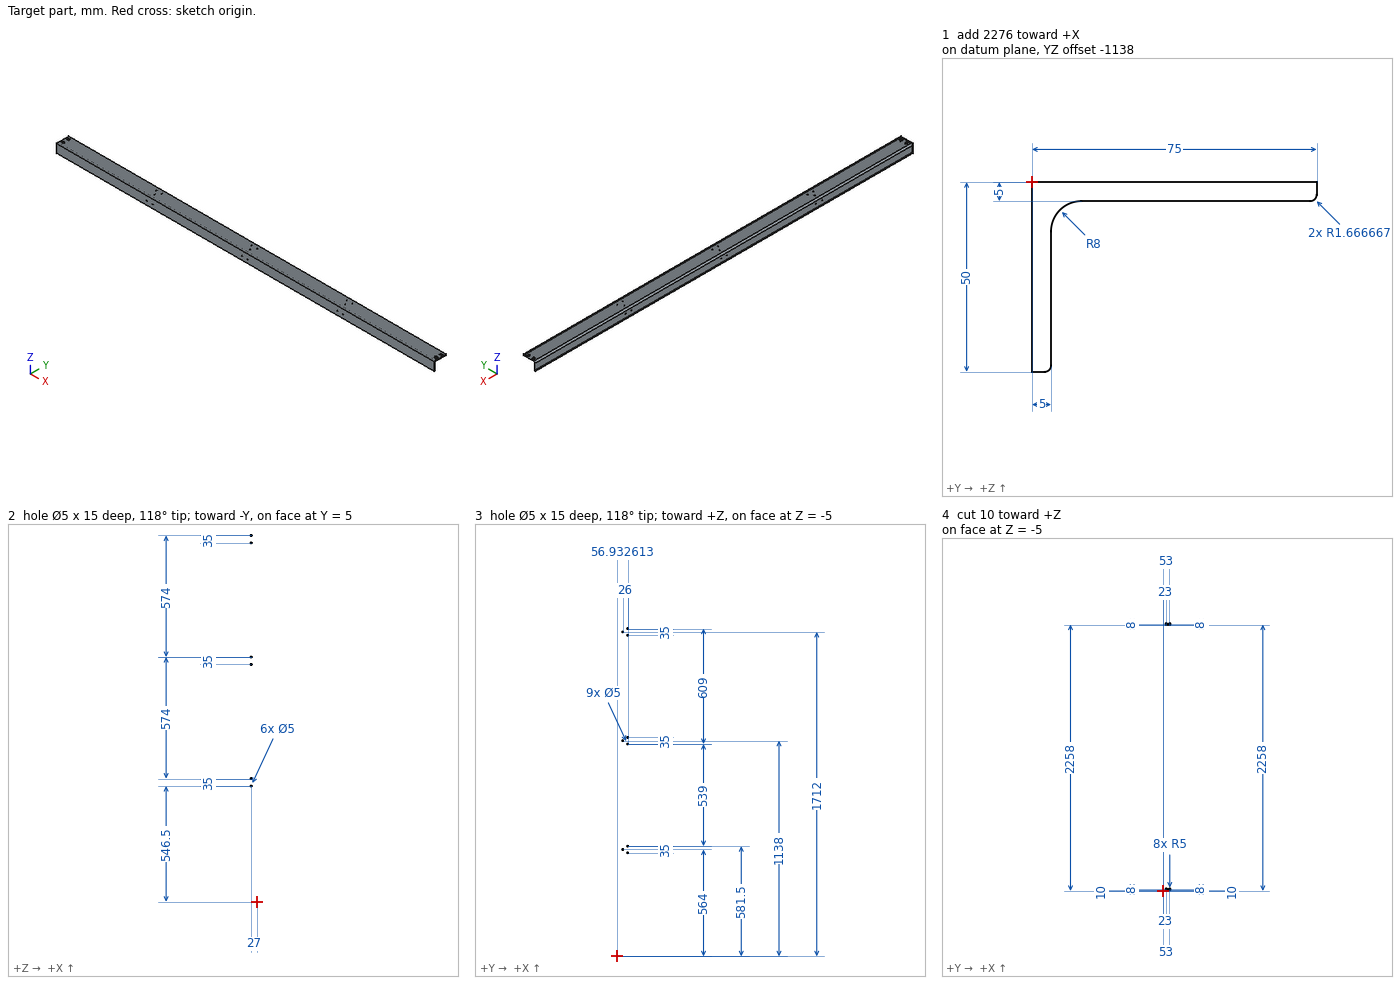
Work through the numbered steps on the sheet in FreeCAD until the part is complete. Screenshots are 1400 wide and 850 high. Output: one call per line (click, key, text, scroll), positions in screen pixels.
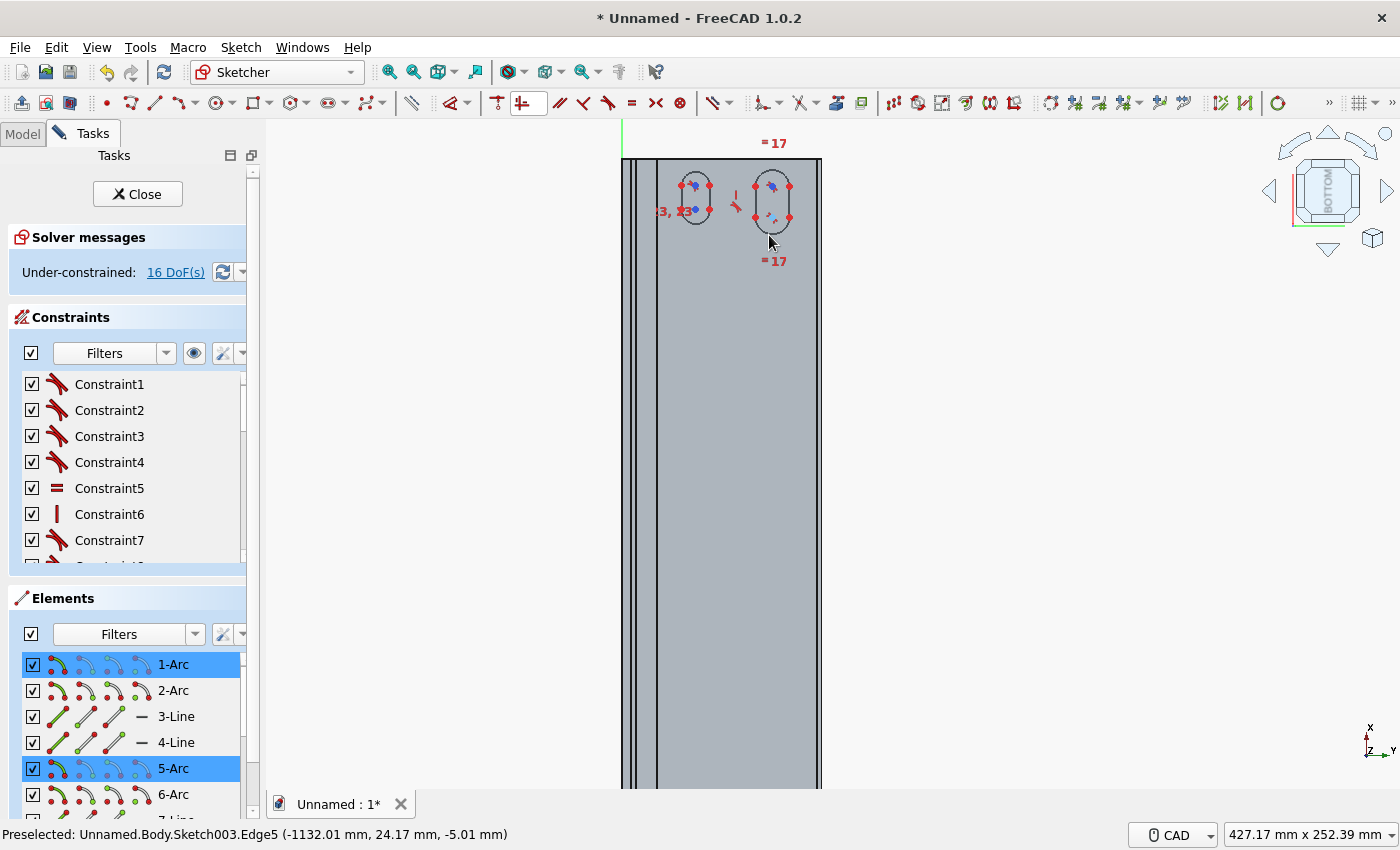
click(763, 231)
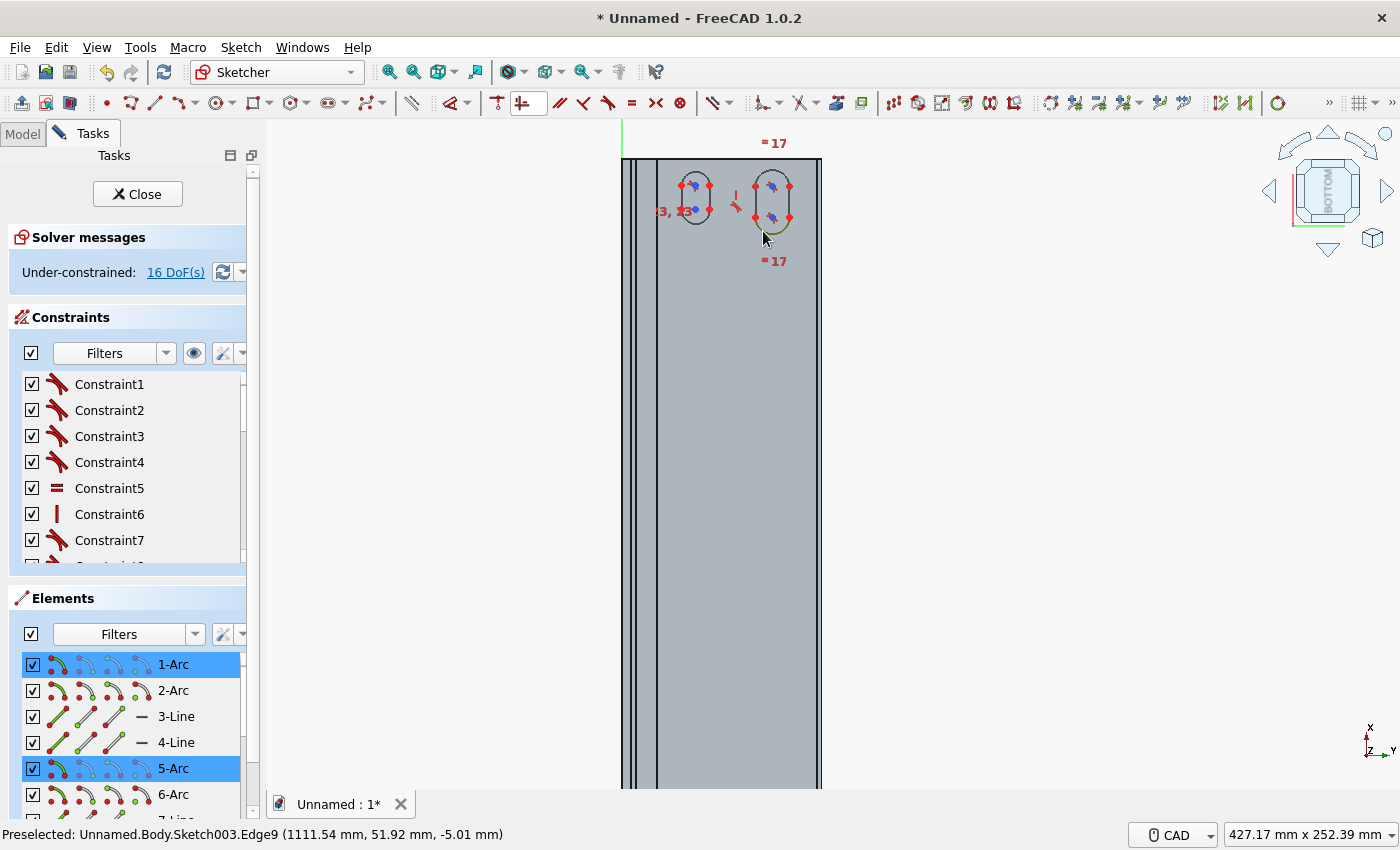
click(688, 221)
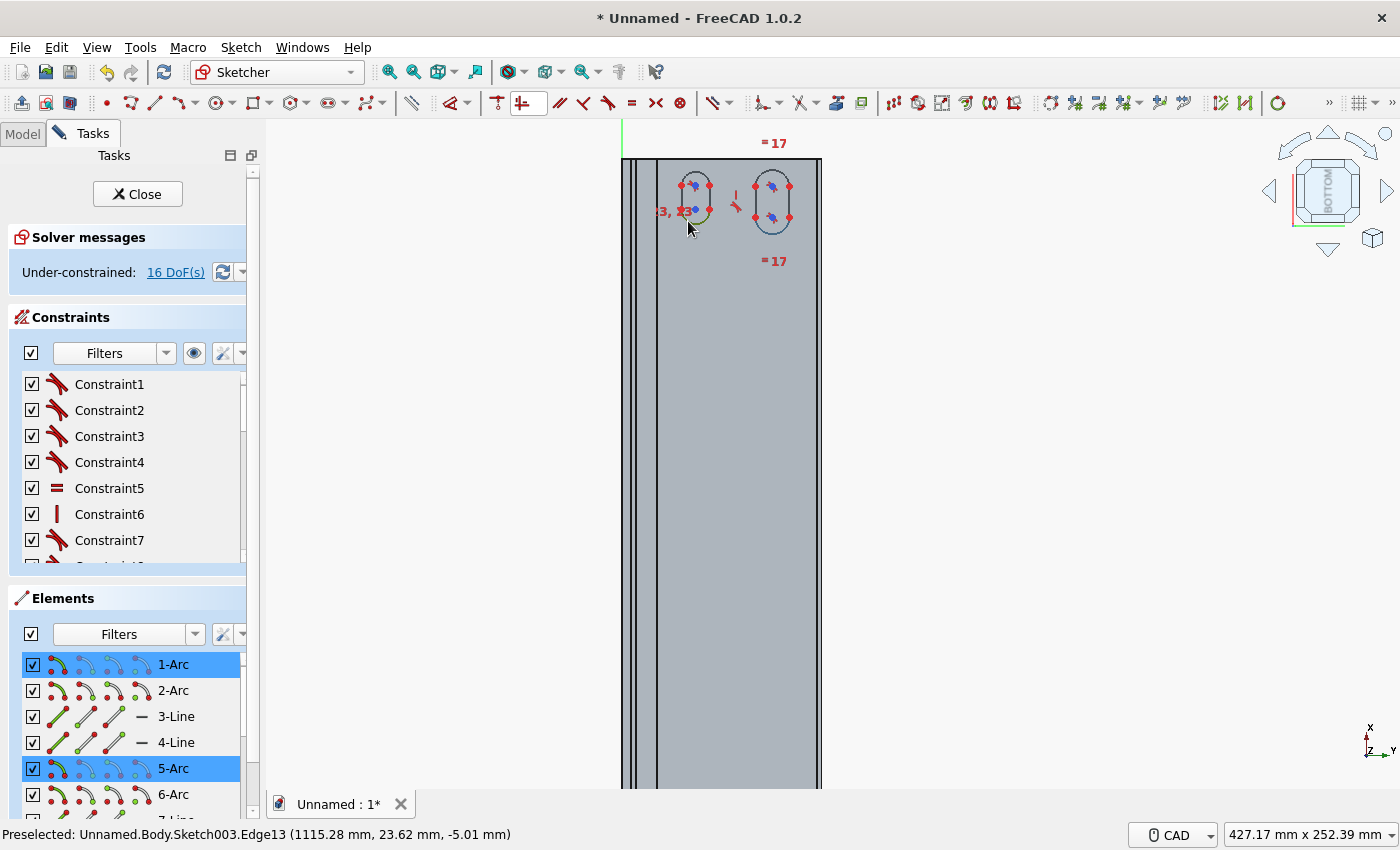
click(632, 104)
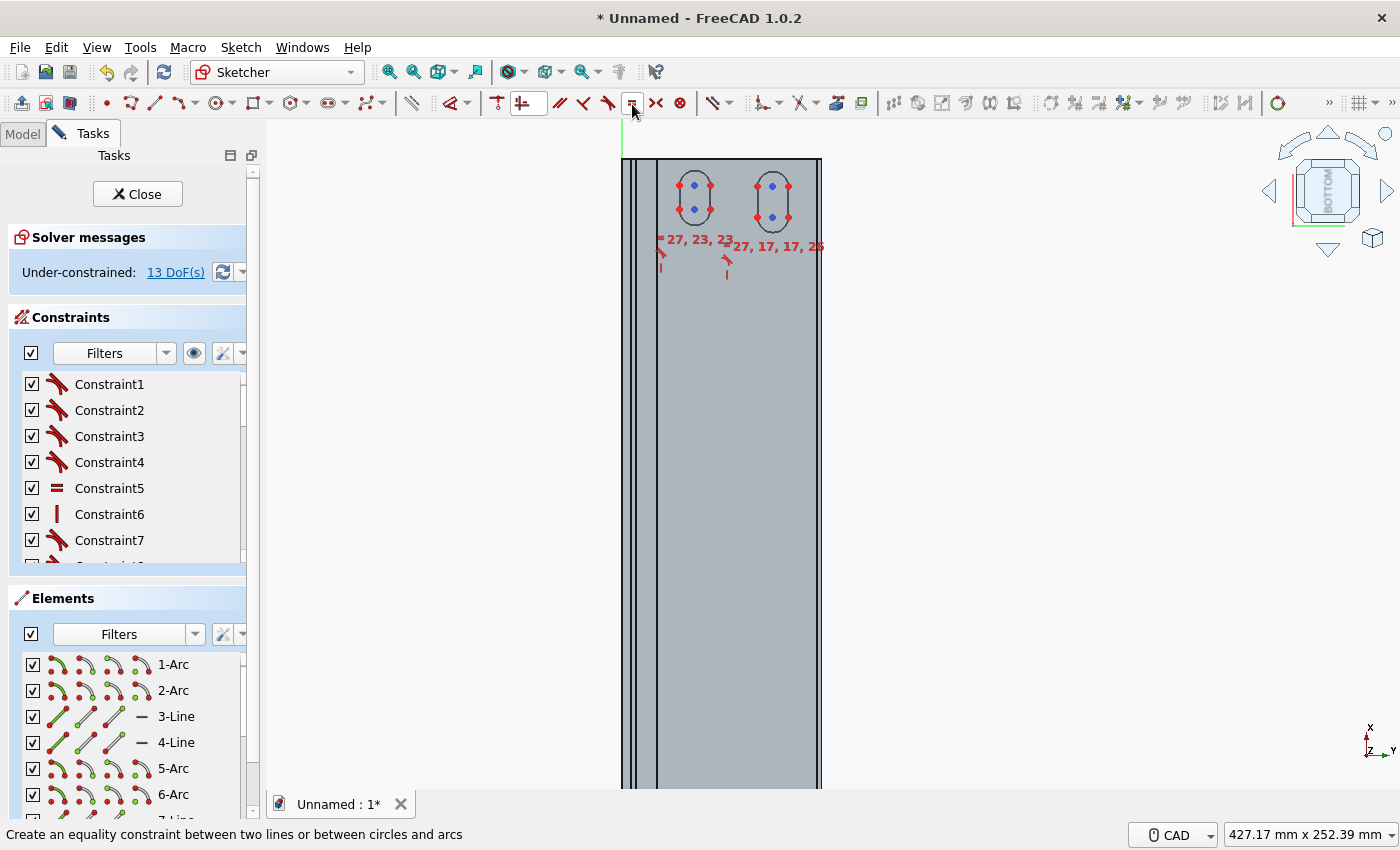
click(450, 104)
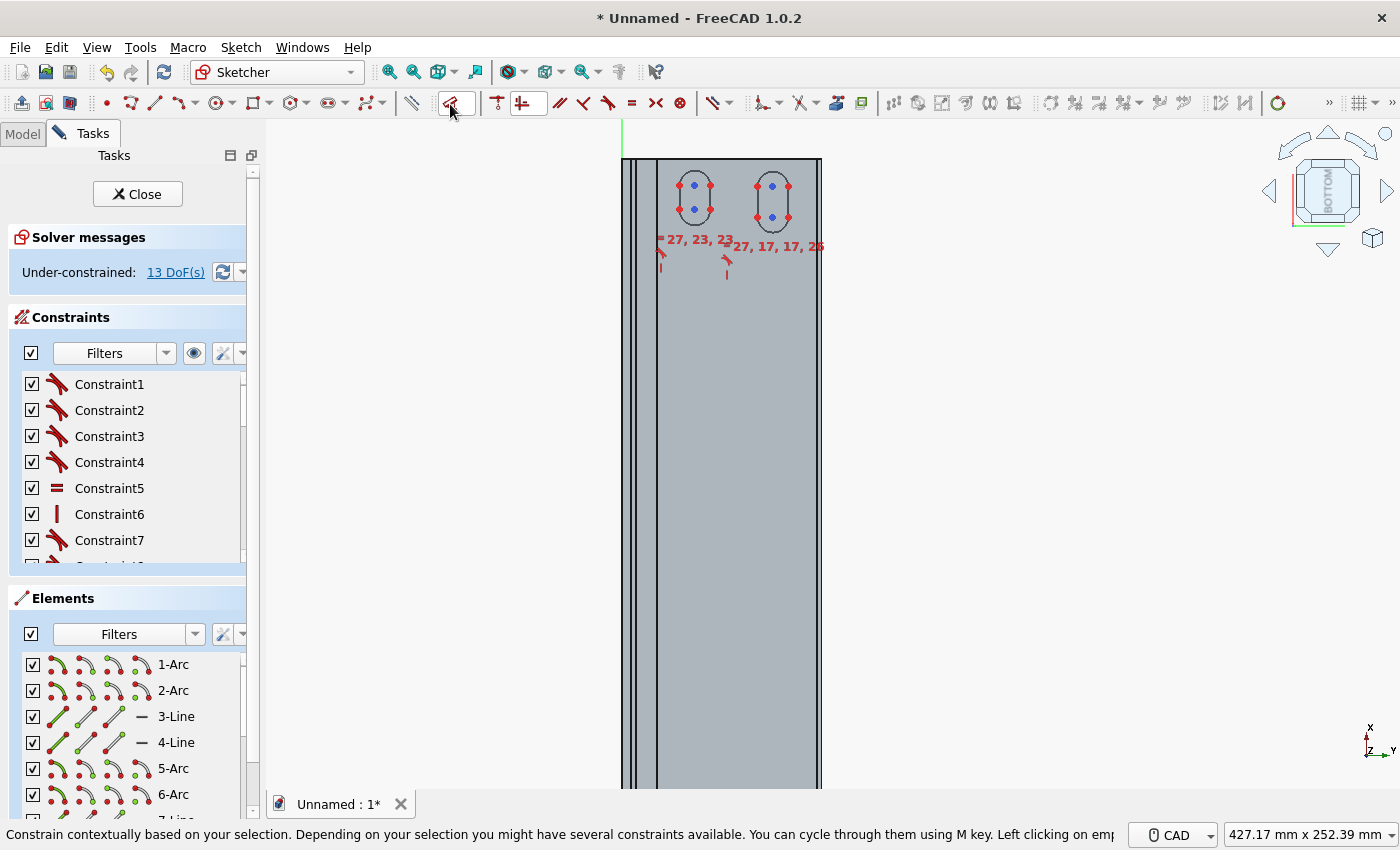
scroll(769, 235, down, 13)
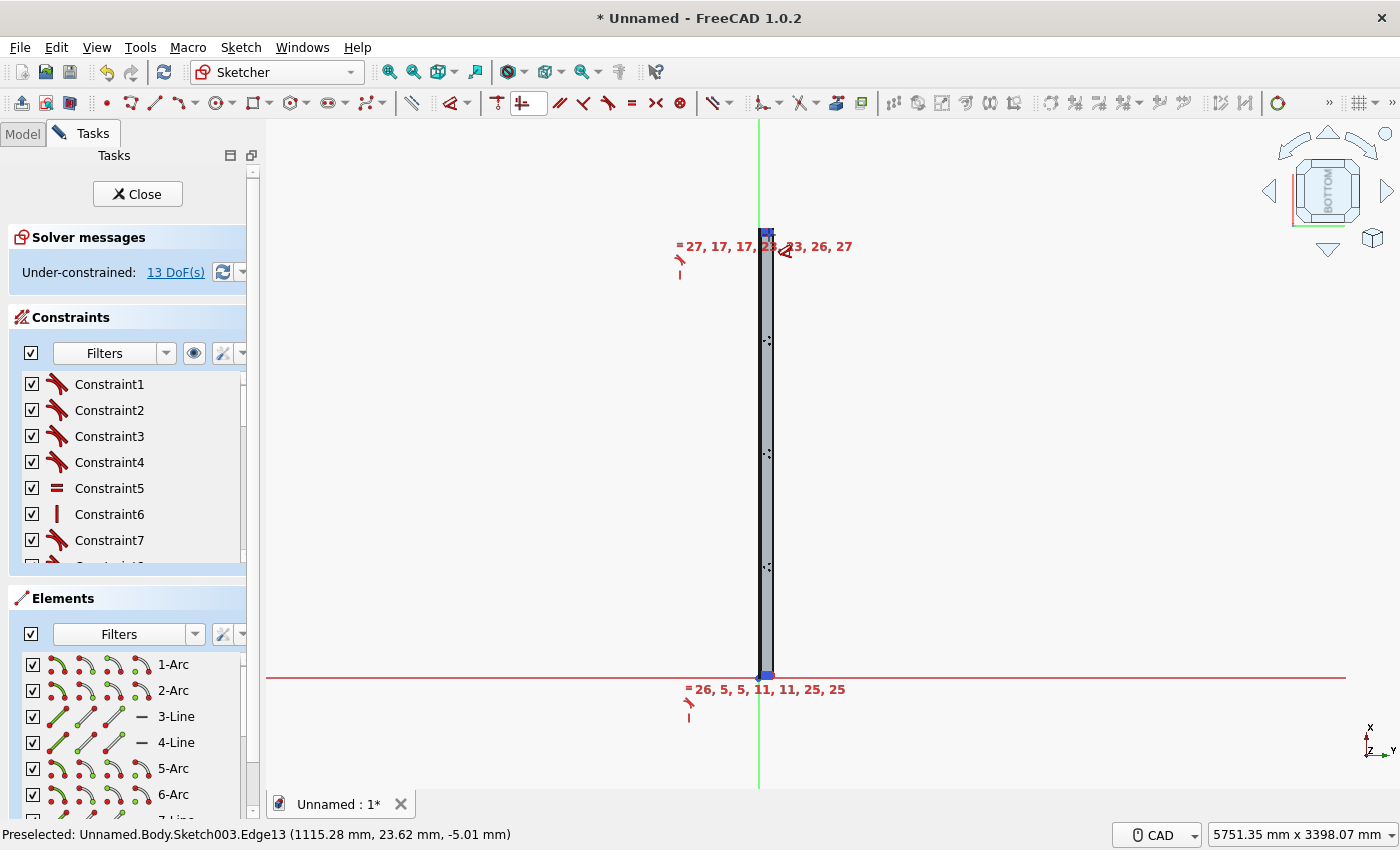
scroll(769, 677, up, 19)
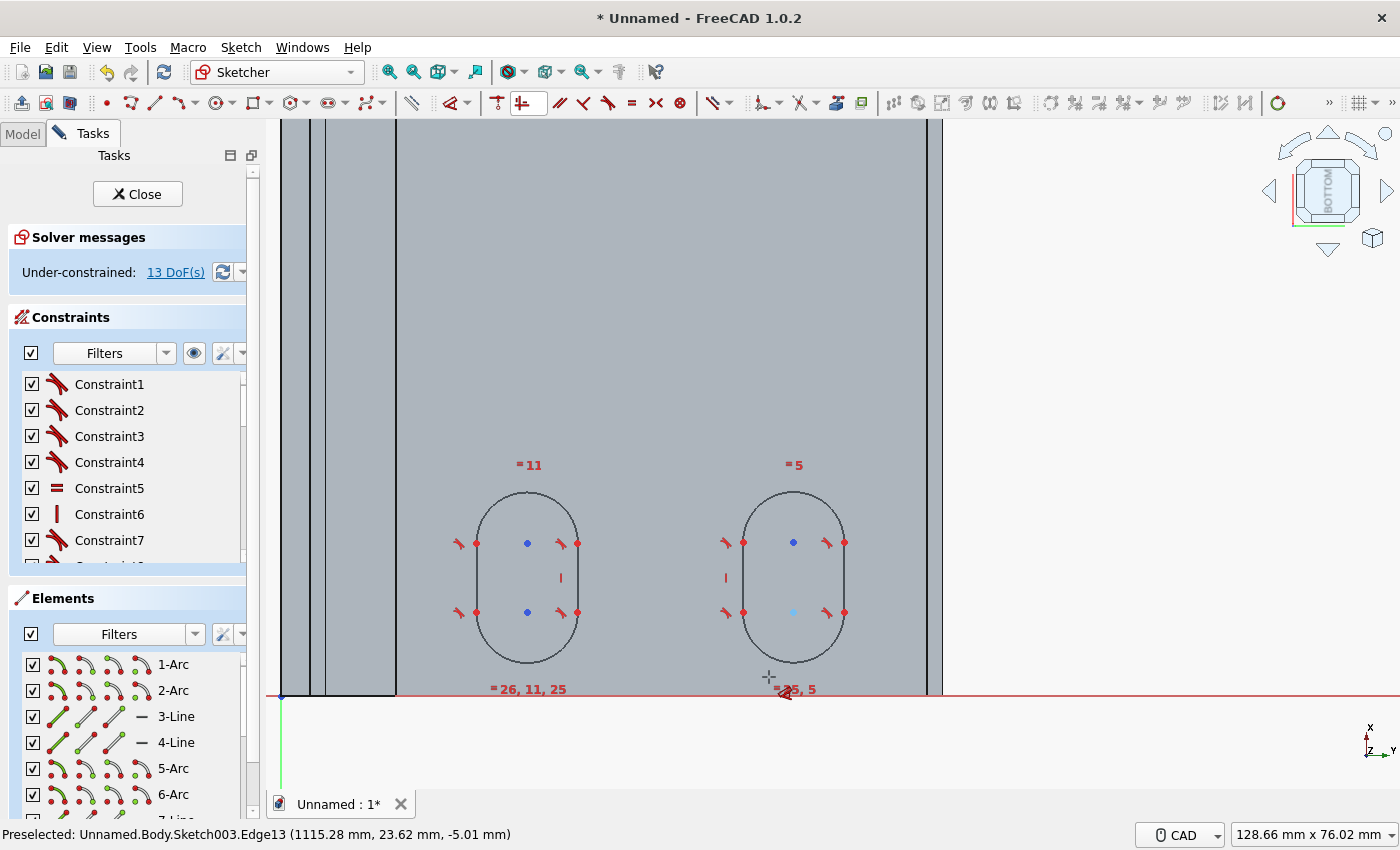
click(764, 653)
click(745, 679)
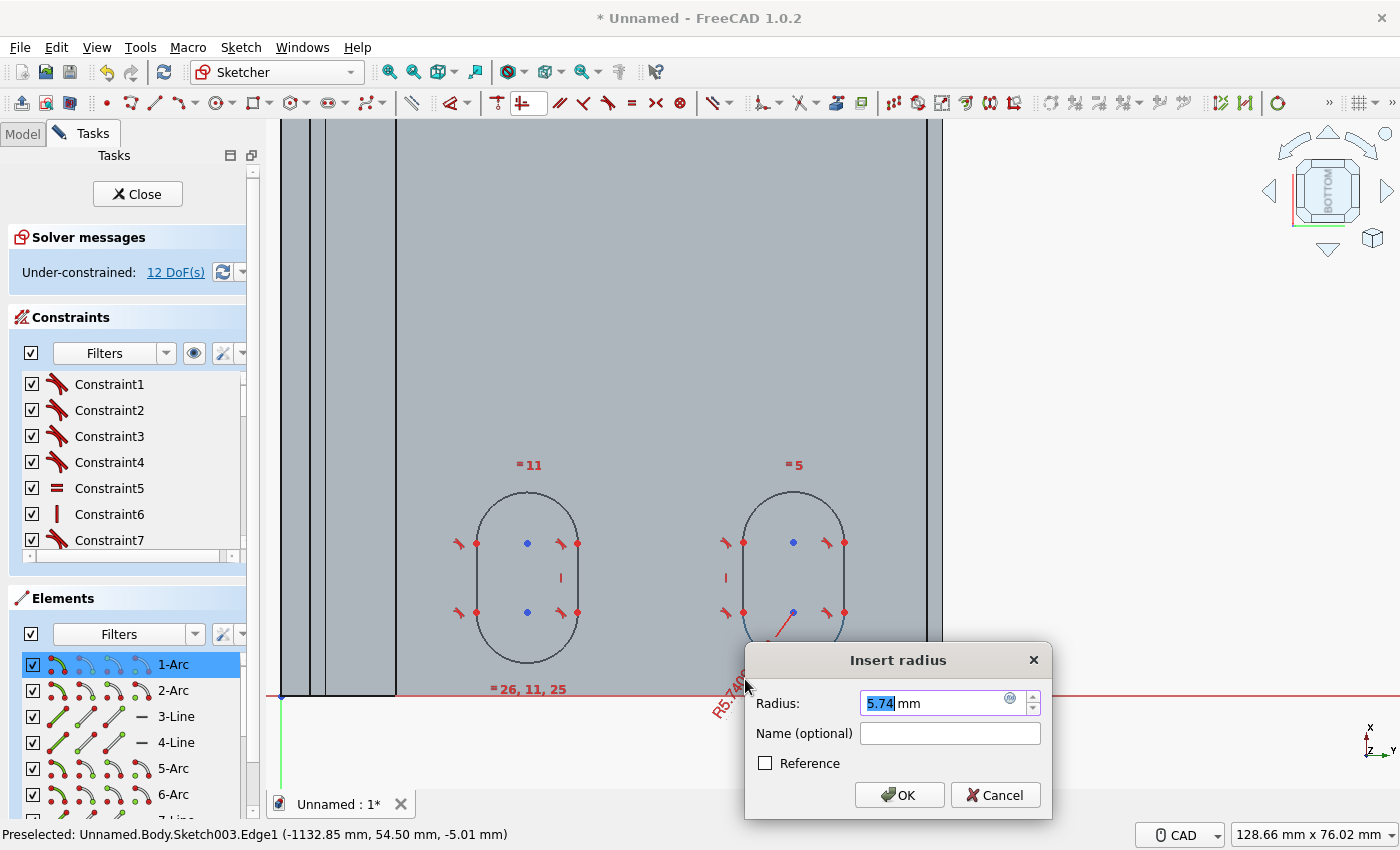
text(5)
key(Return)